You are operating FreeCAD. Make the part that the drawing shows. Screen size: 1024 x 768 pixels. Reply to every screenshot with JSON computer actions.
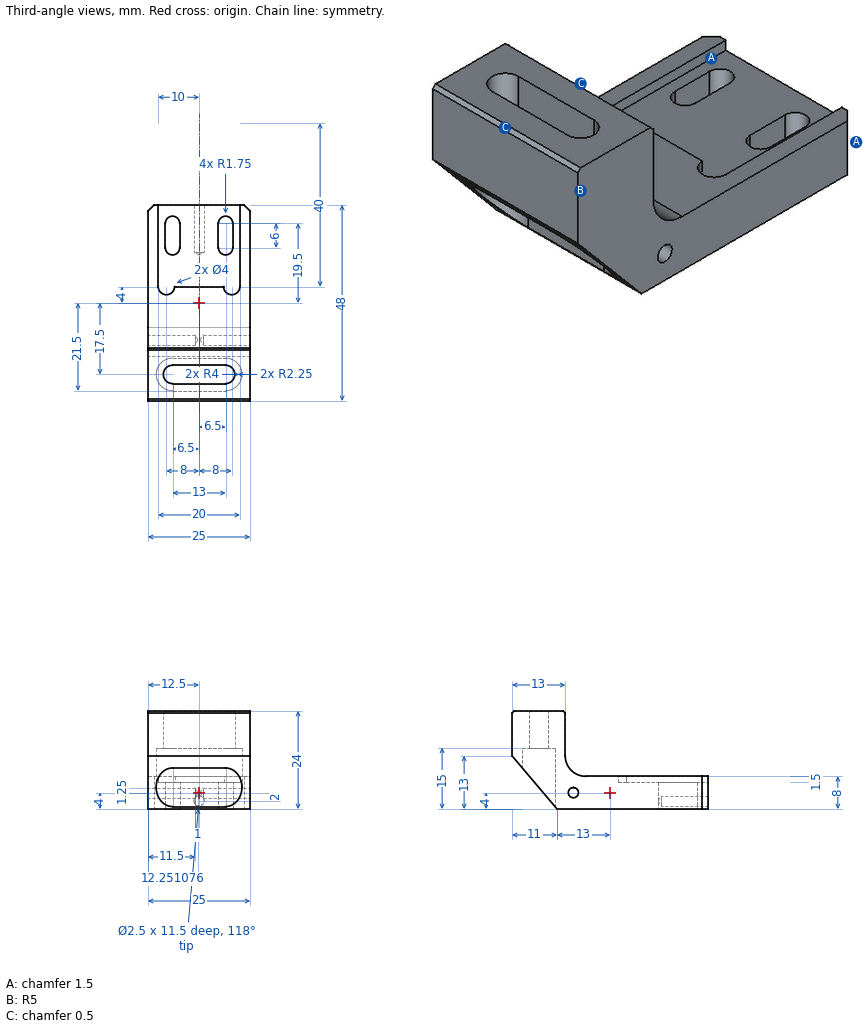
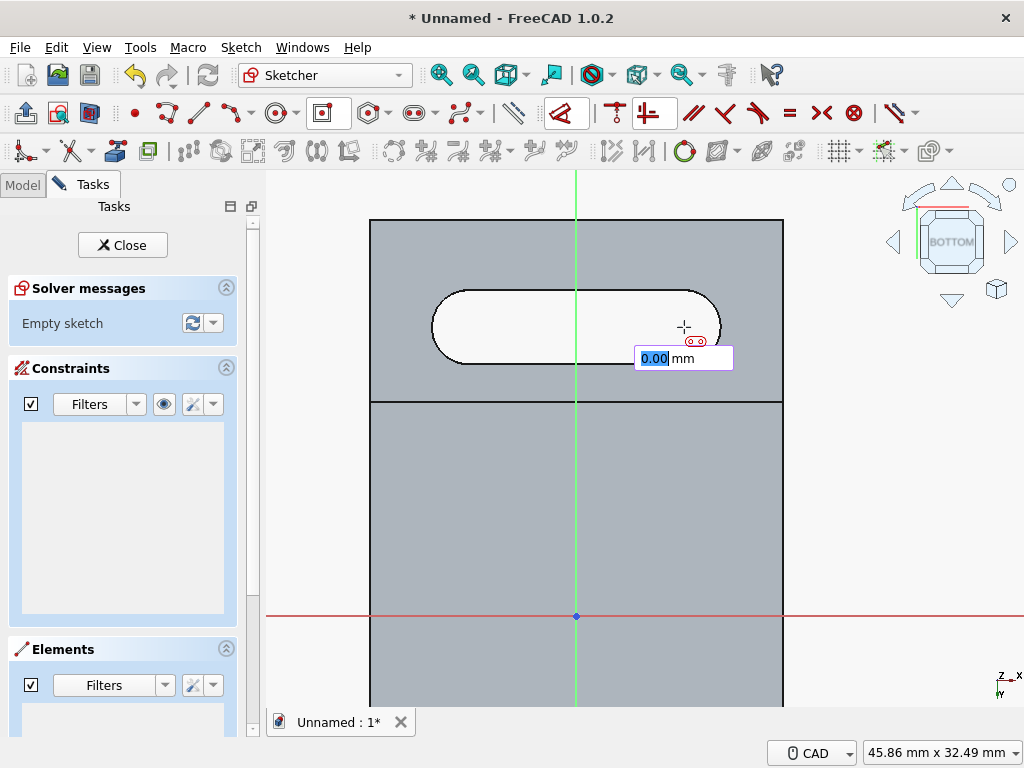
{"action": "left_click", "coordinate": [544, 393]}
{"action": "key", "text": "Escape"}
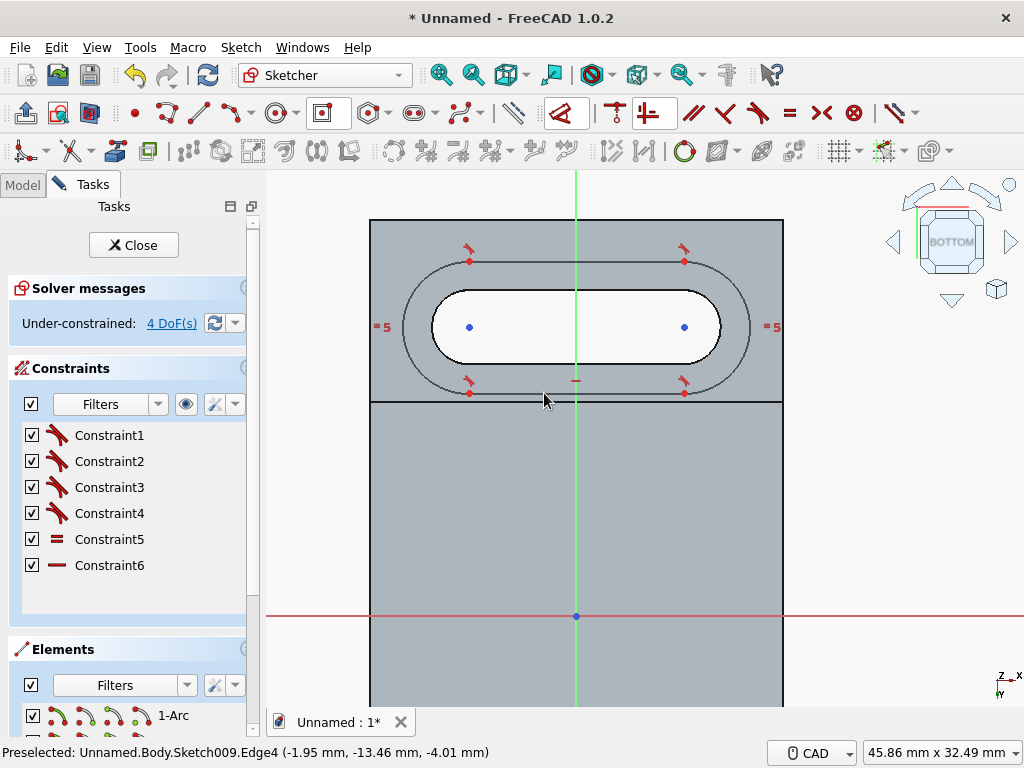
{"action": "left_click", "coordinate": [416, 289]}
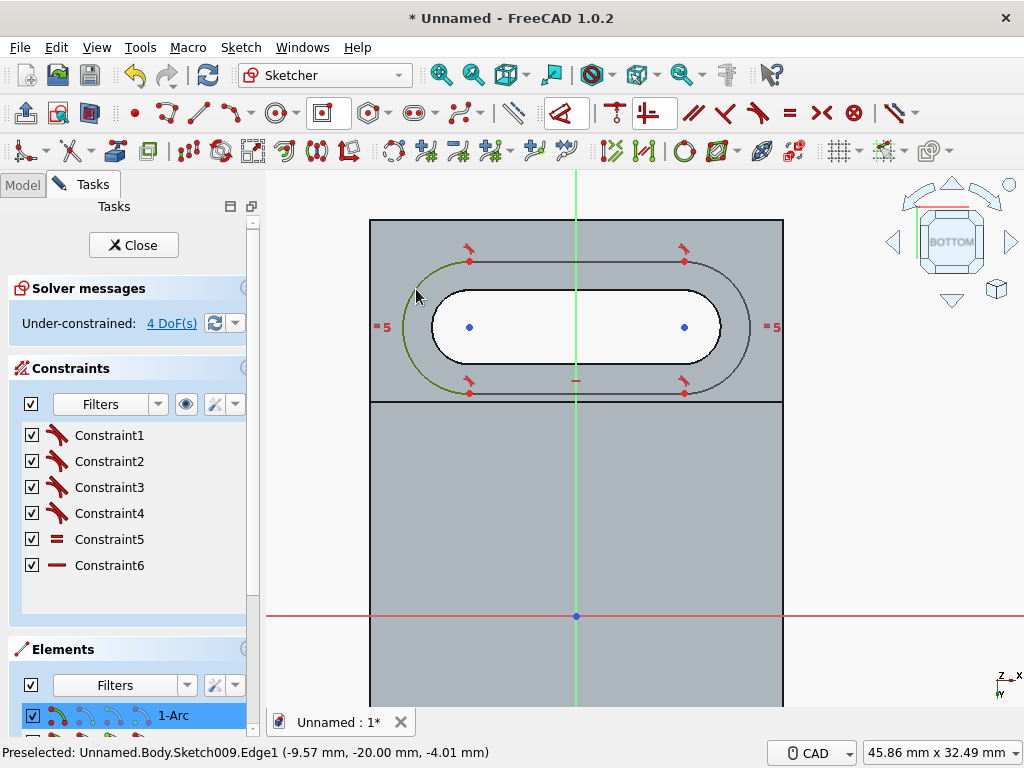
{"action": "key", "text": "k r"}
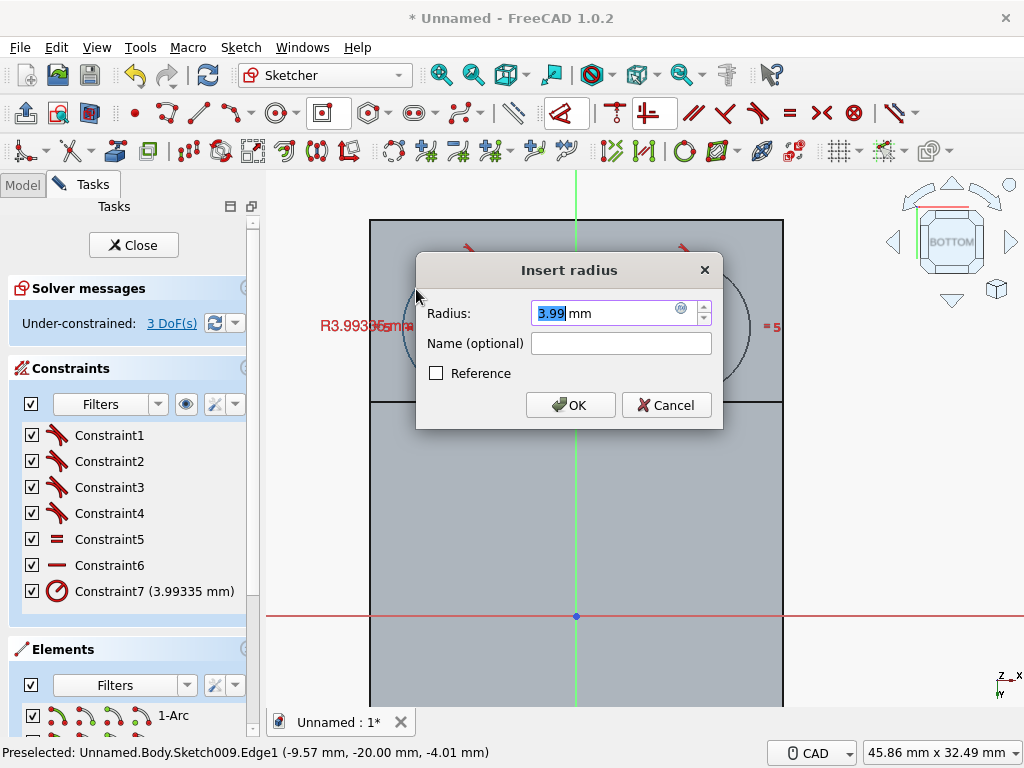
{"action": "type", "text": "4"}
{"action": "key", "text": "Return"}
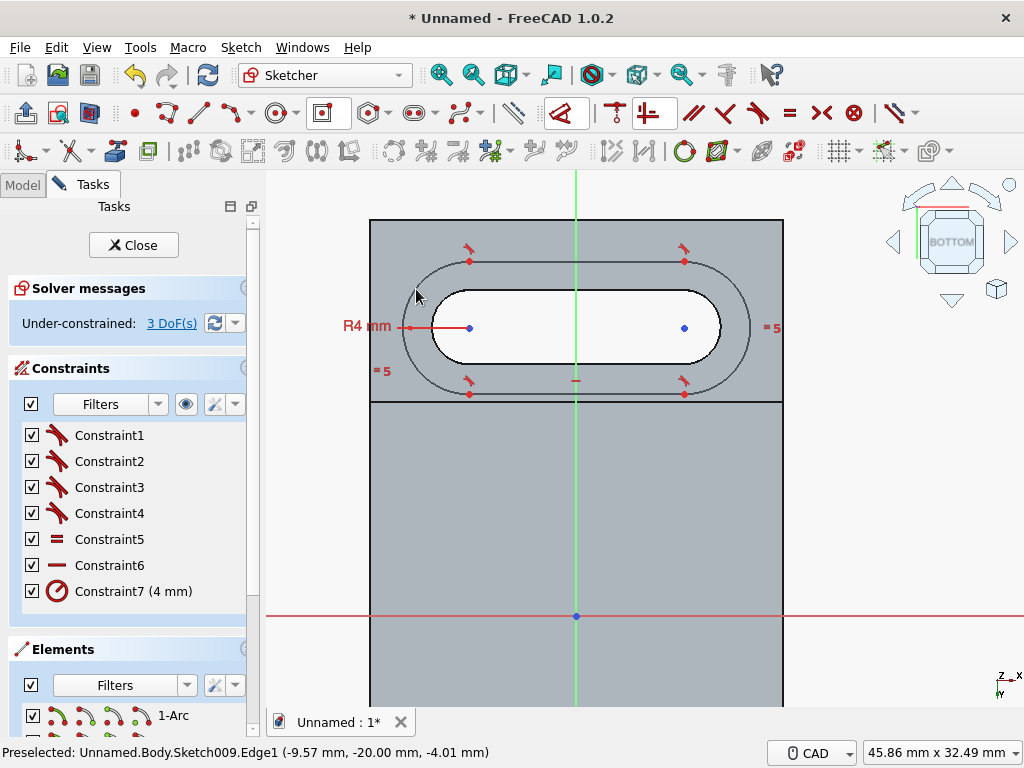
{"action": "left_click", "coordinate": [534, 262]}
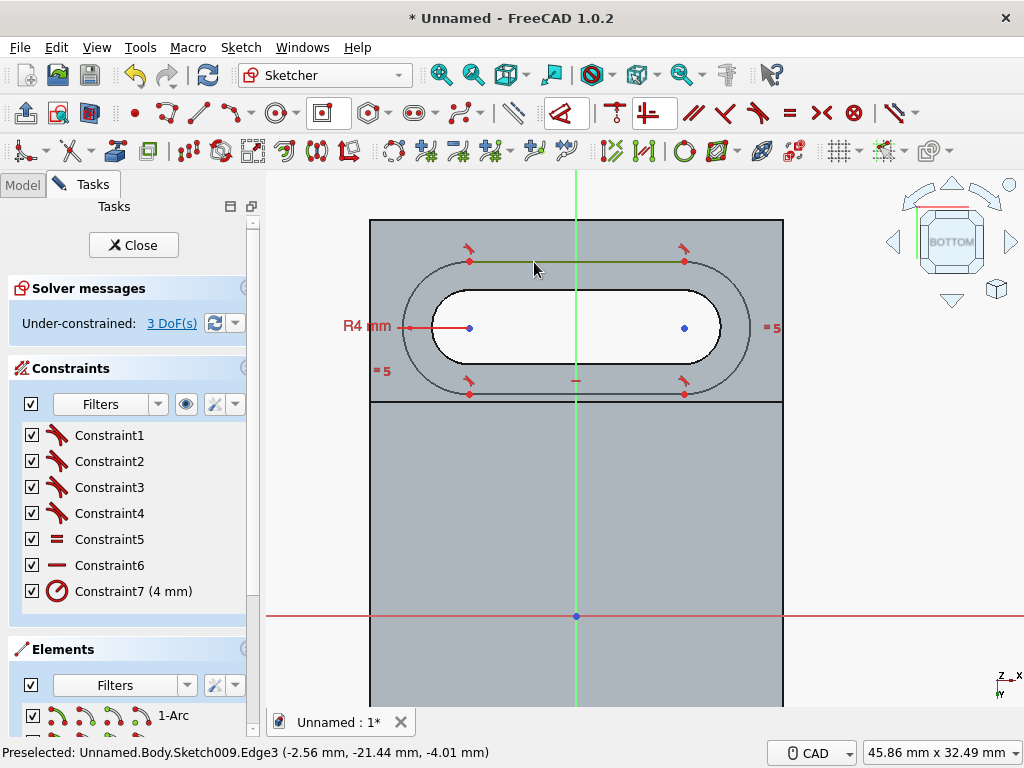
{"action": "key", "text": "l"}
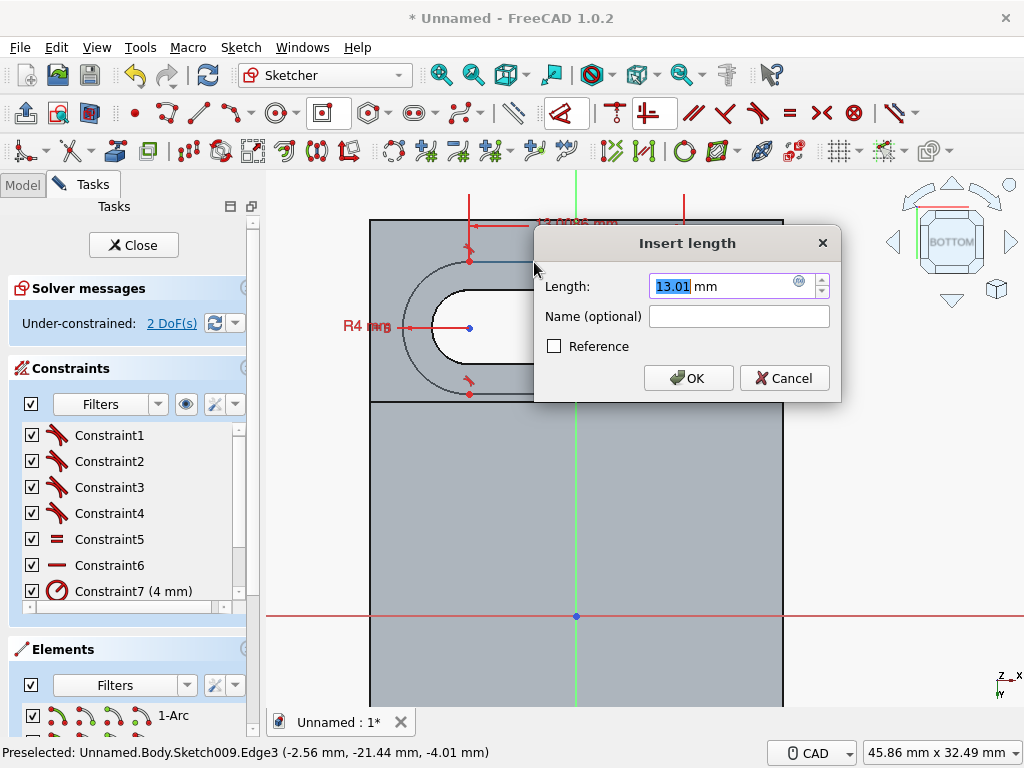
{"action": "type", "text": "13"}
{"action": "key", "text": "Return"}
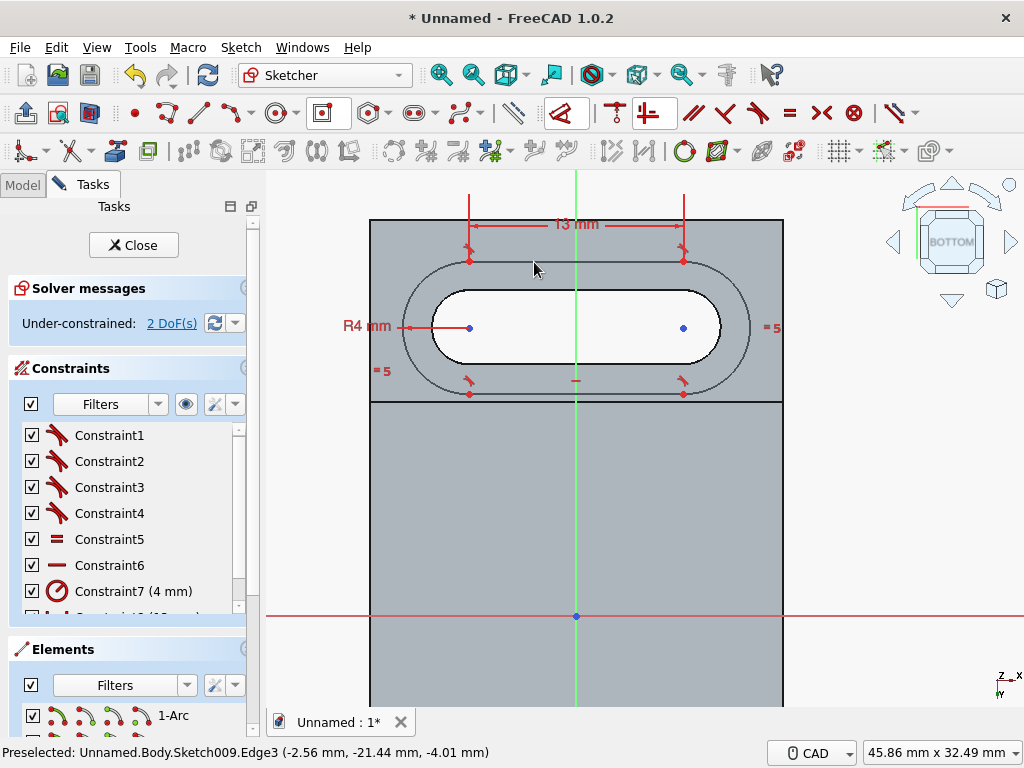
{"action": "left_click", "coordinate": [469, 262]}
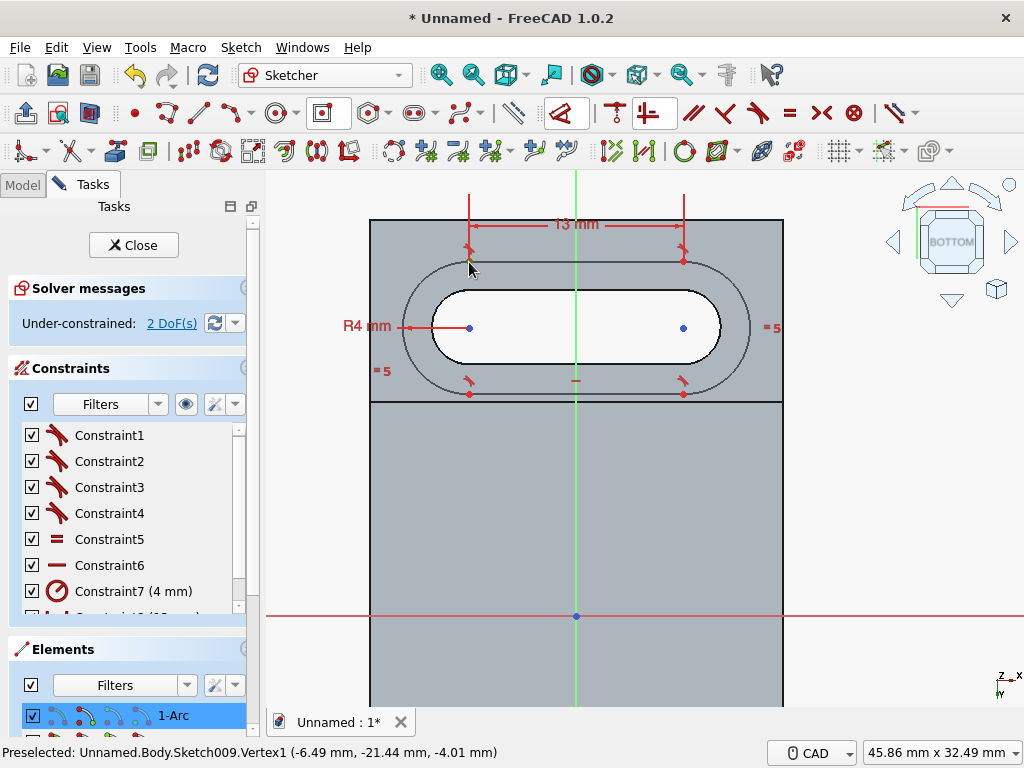
{"action": "key", "text": "l"}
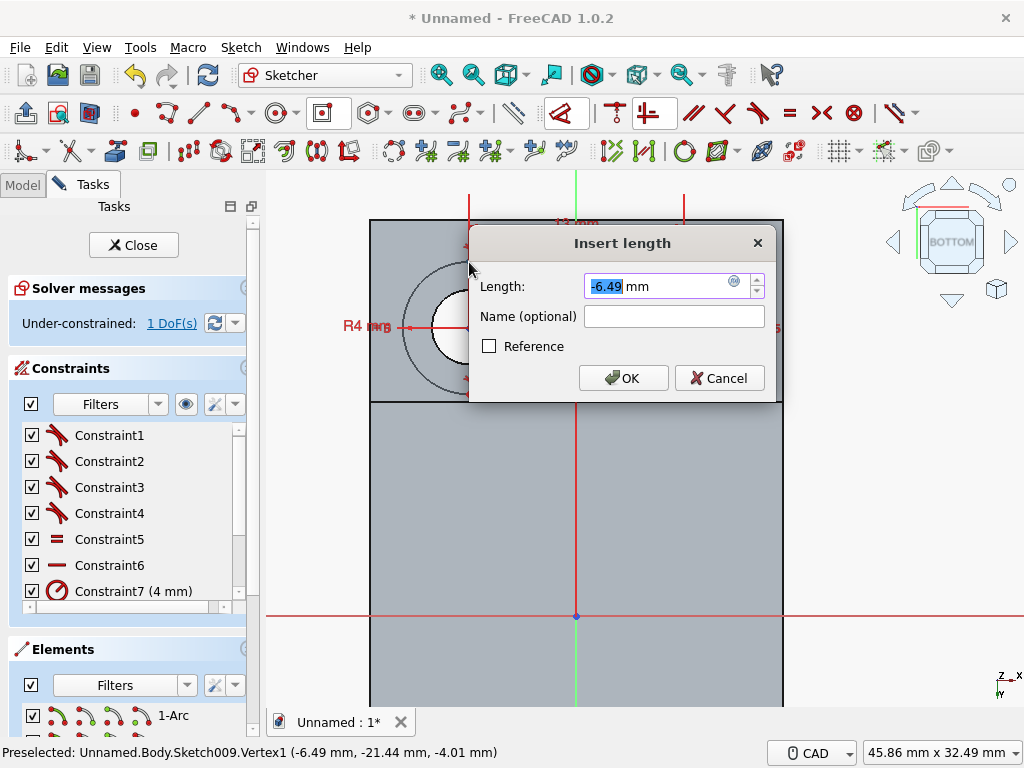
{"action": "type", "text": "-6.5"}
{"action": "key", "text": "Return"}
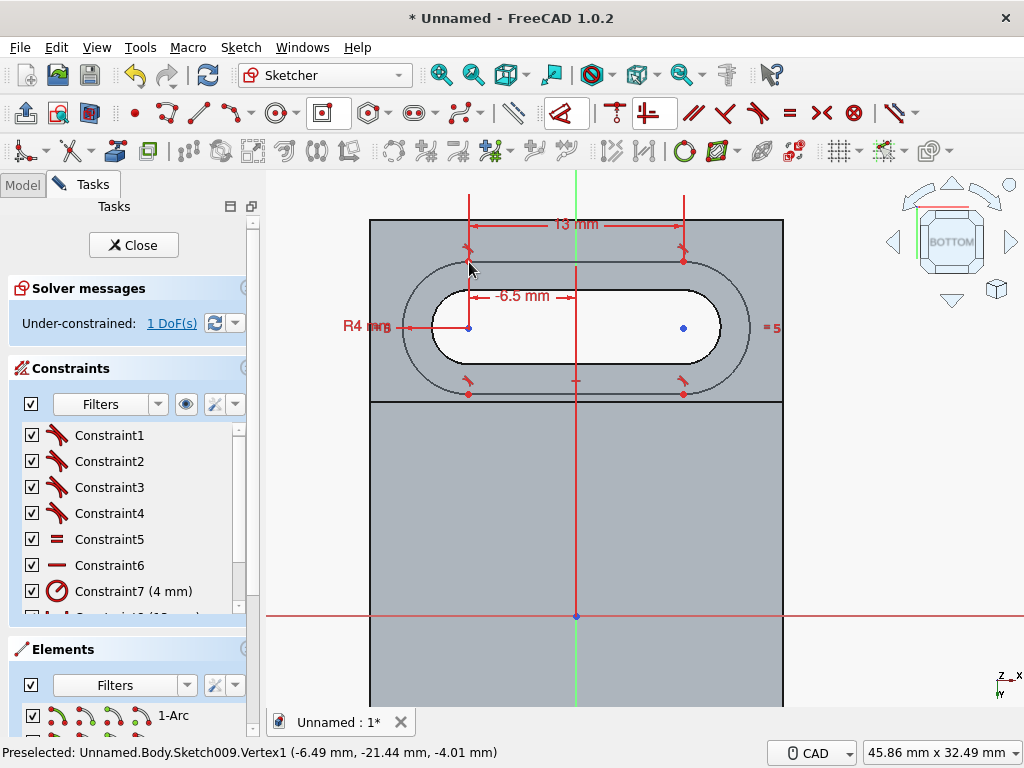
{"action": "left_click", "coordinate": [469, 262]}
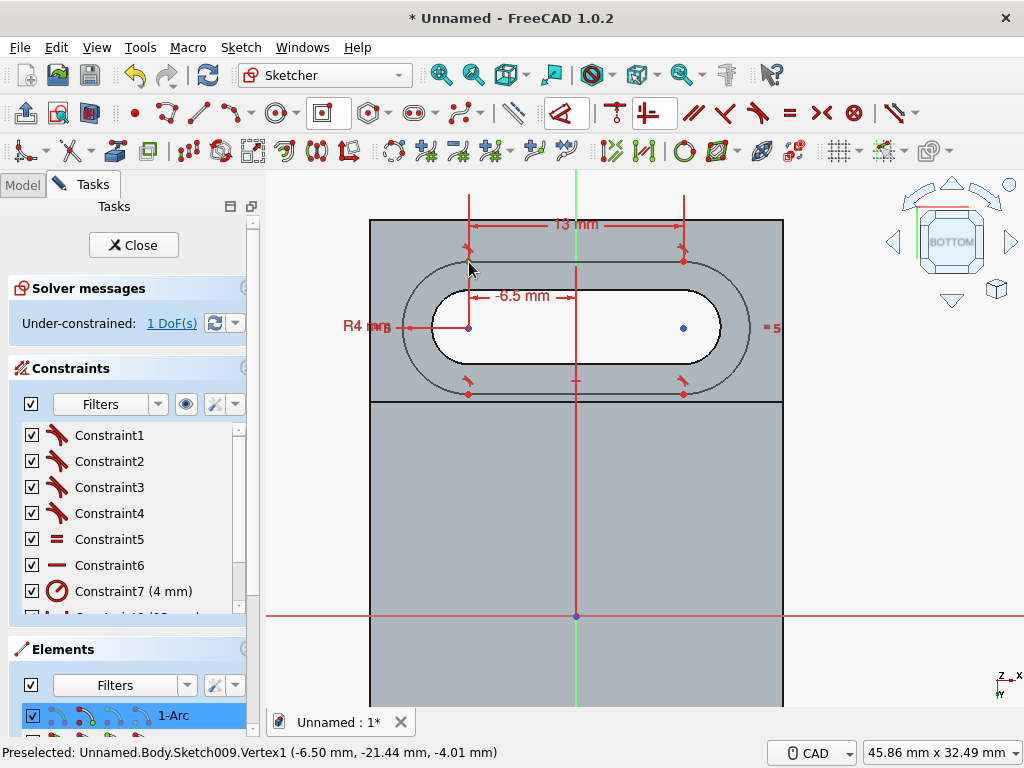
{"action": "key", "text": "i"}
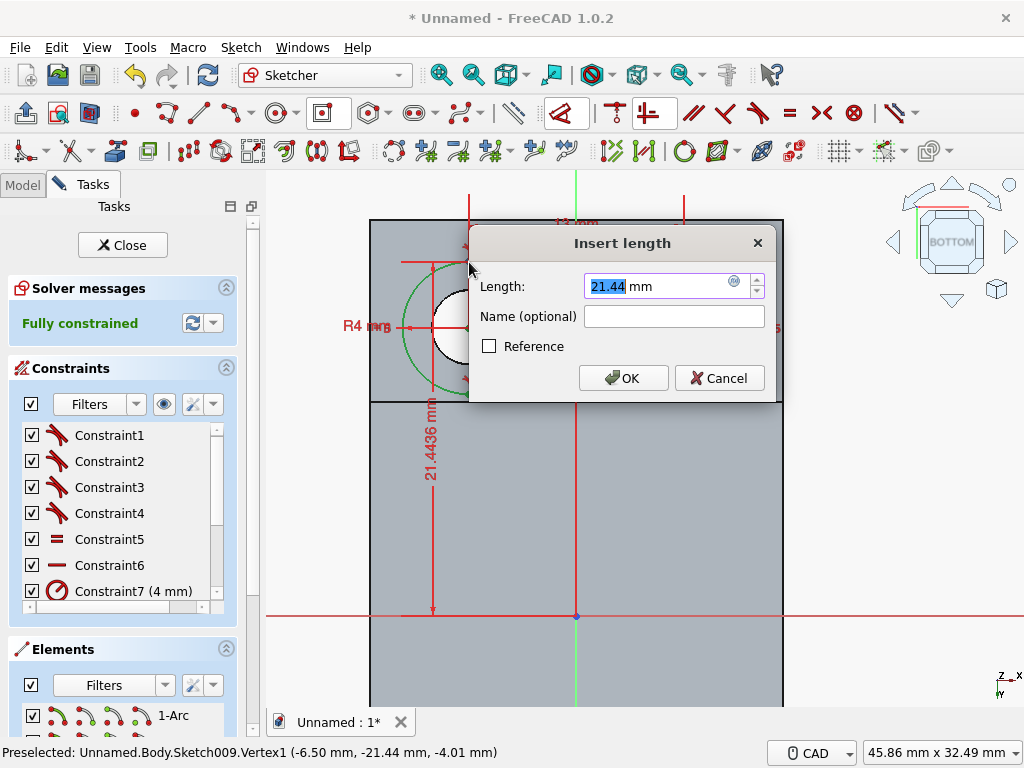
{"action": "type", "text": "21.5"}
{"action": "key", "text": "Return"}